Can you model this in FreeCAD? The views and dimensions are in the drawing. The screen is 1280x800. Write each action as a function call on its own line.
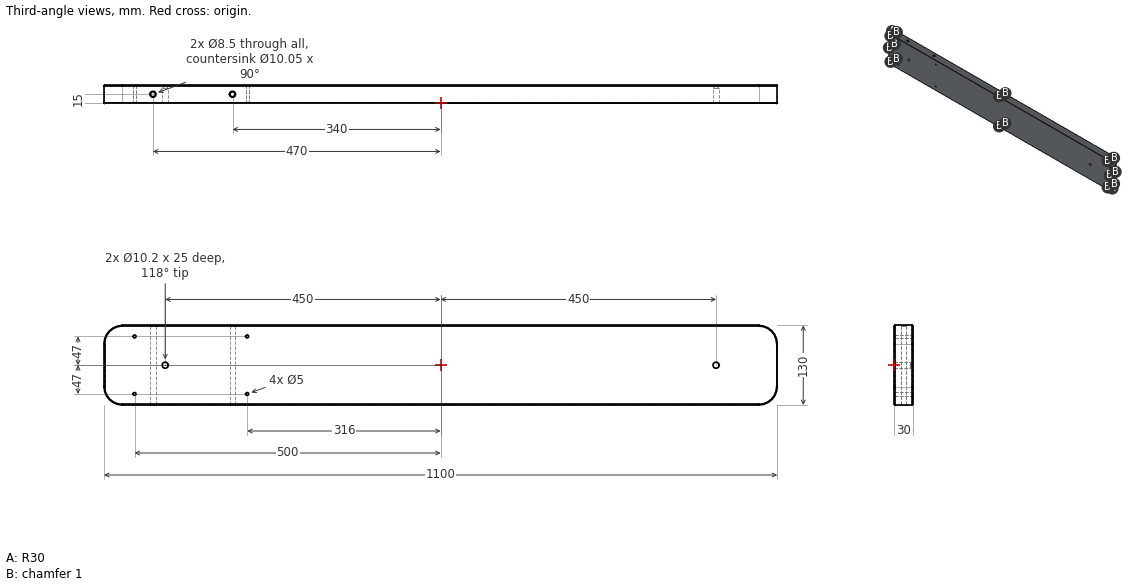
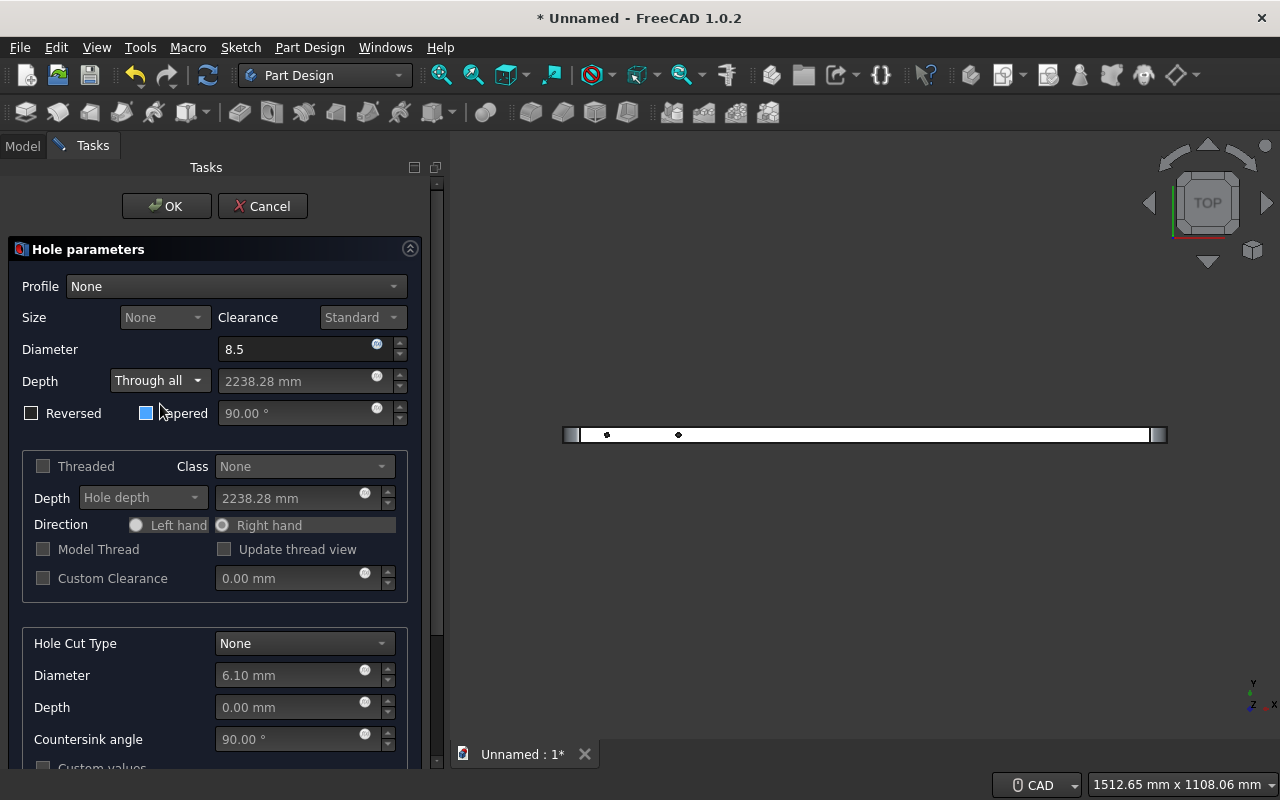
click(306, 644)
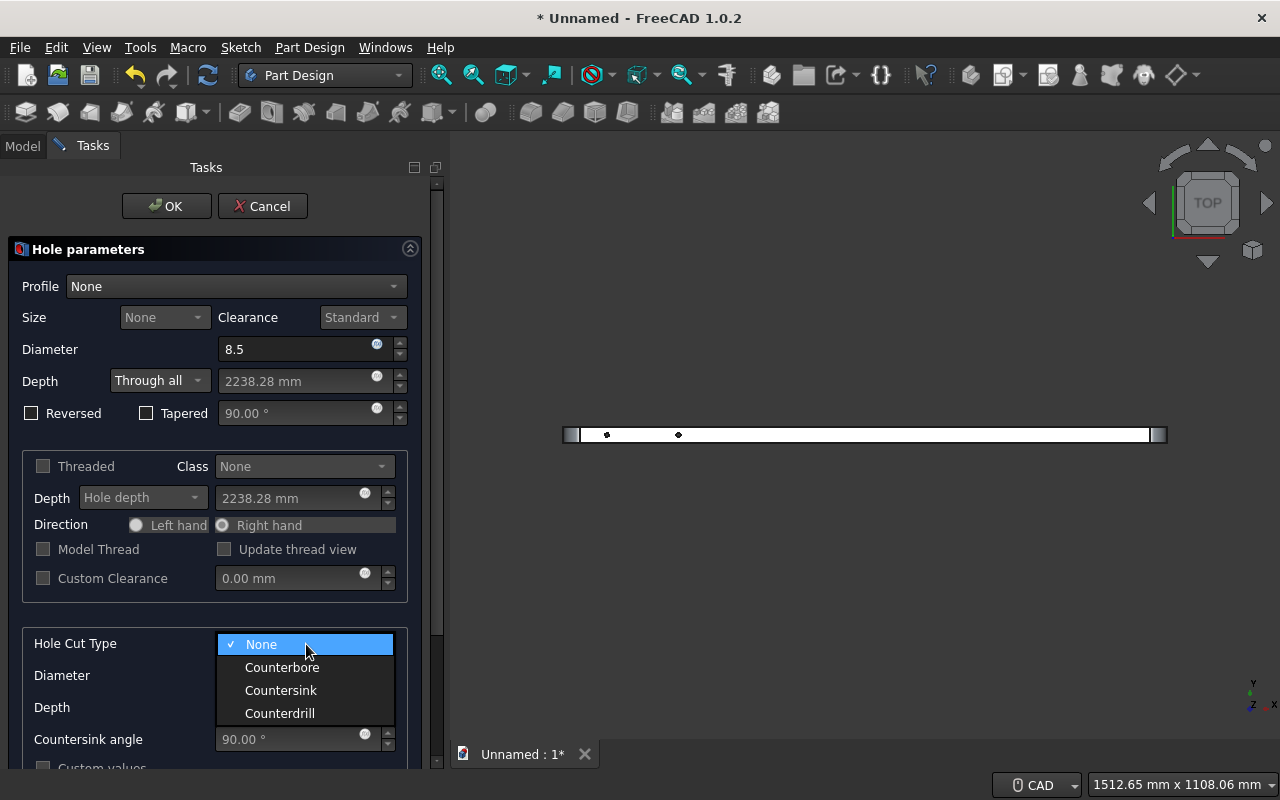
click(304, 690)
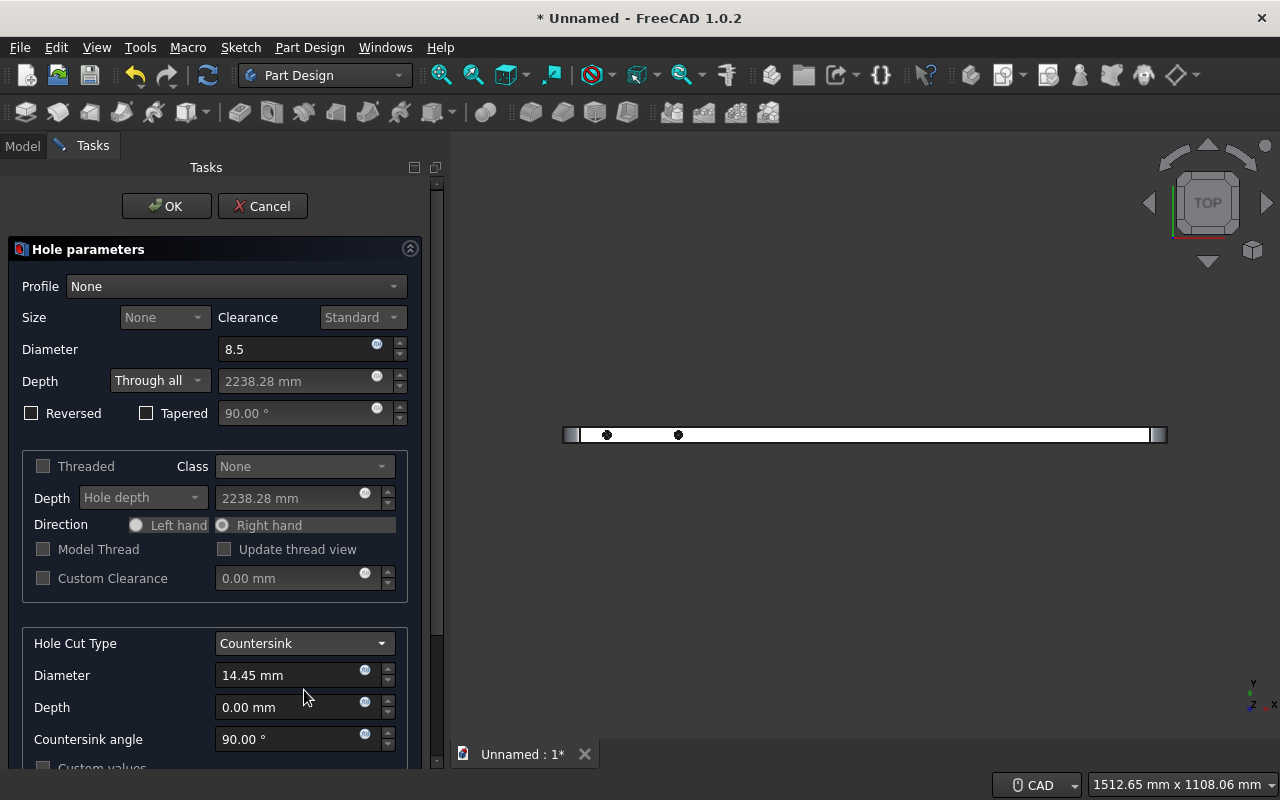
triple_click(298, 675)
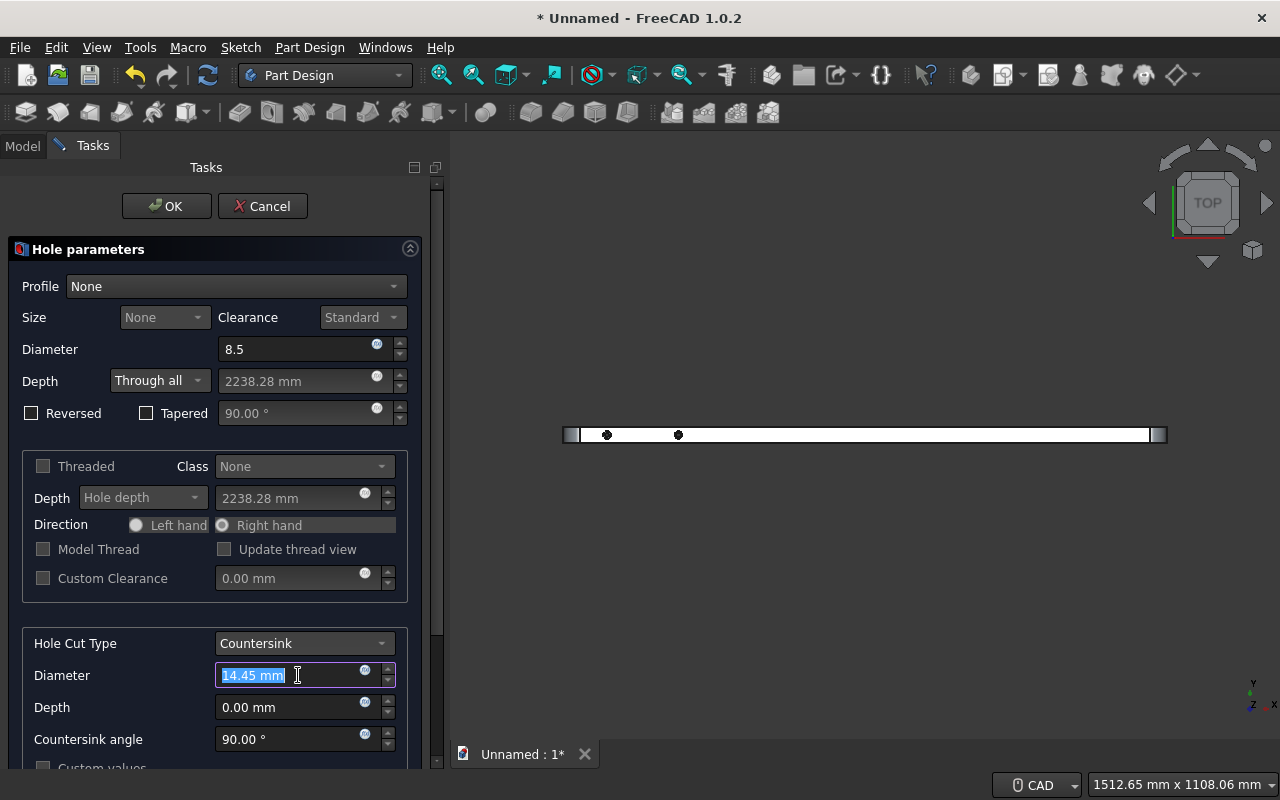
text(10.05)
key(Tab)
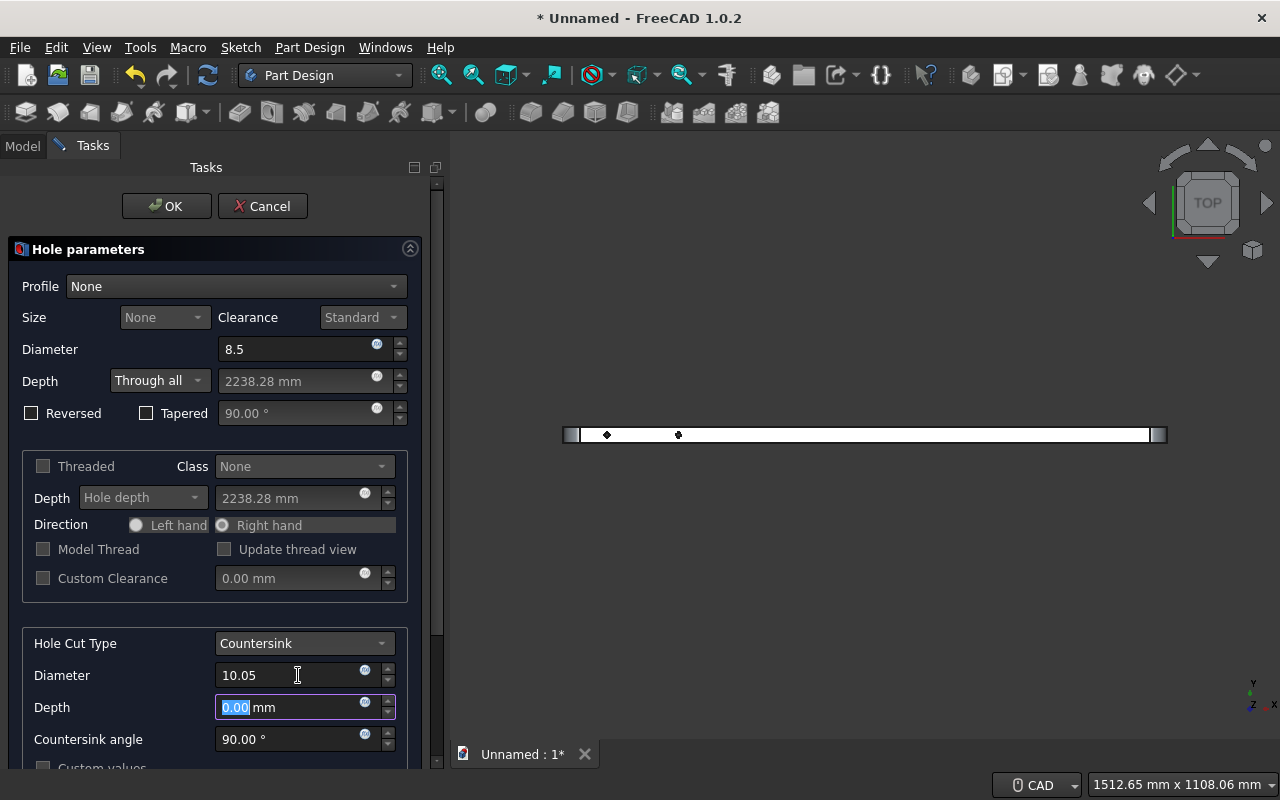
click(167, 206)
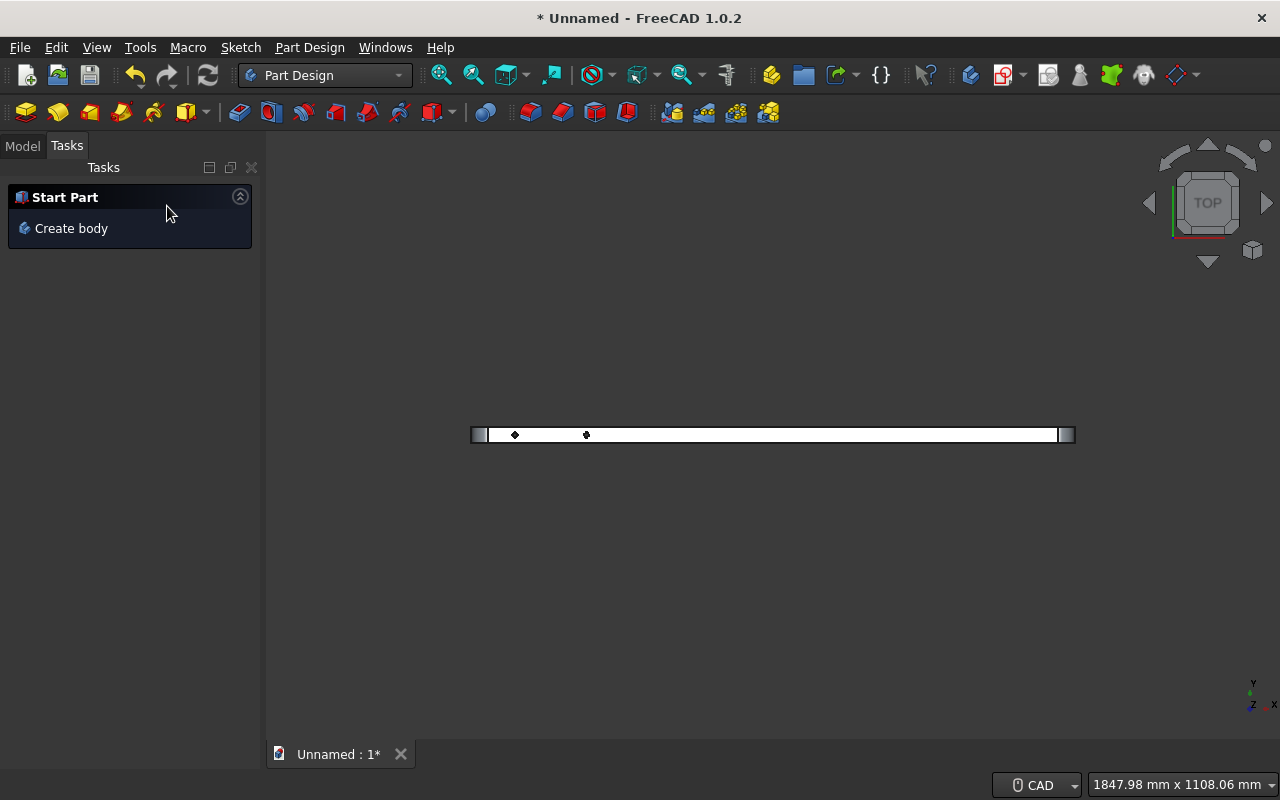
key(0)